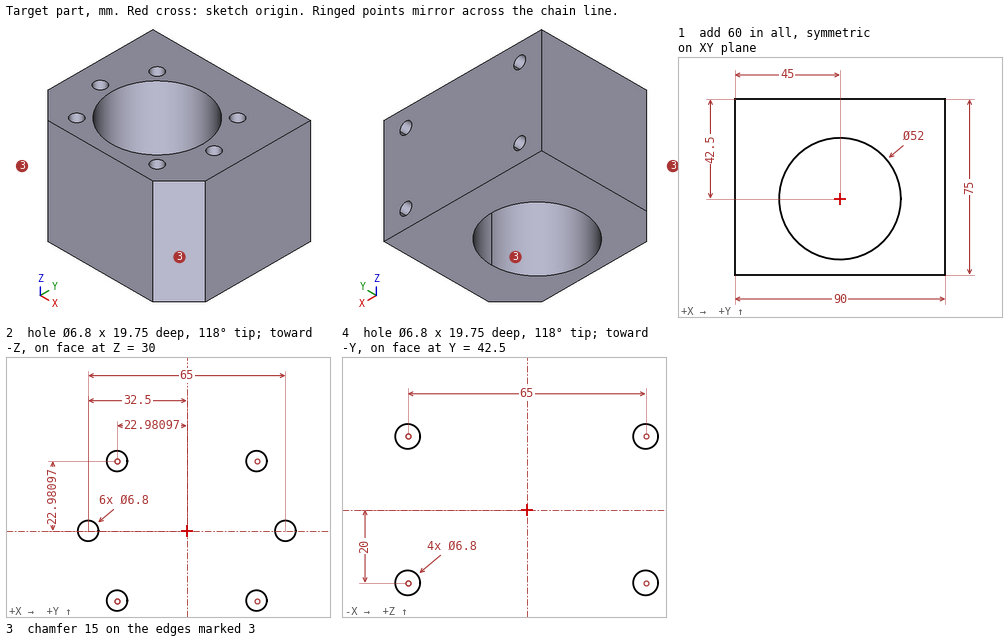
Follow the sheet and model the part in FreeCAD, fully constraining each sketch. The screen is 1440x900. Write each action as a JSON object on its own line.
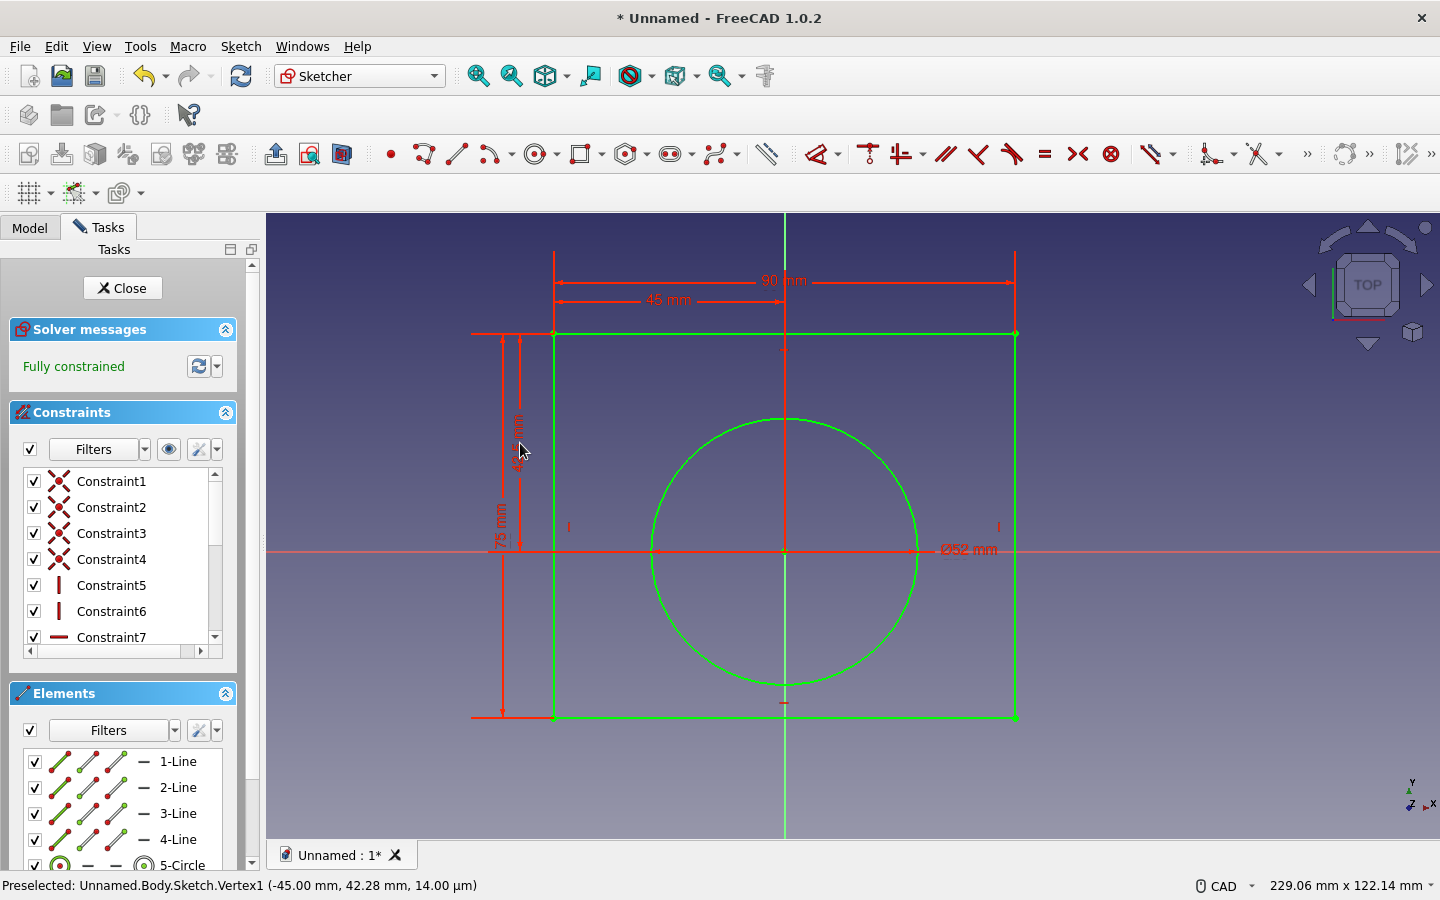
{"action": "left_click", "coordinate": [123, 288]}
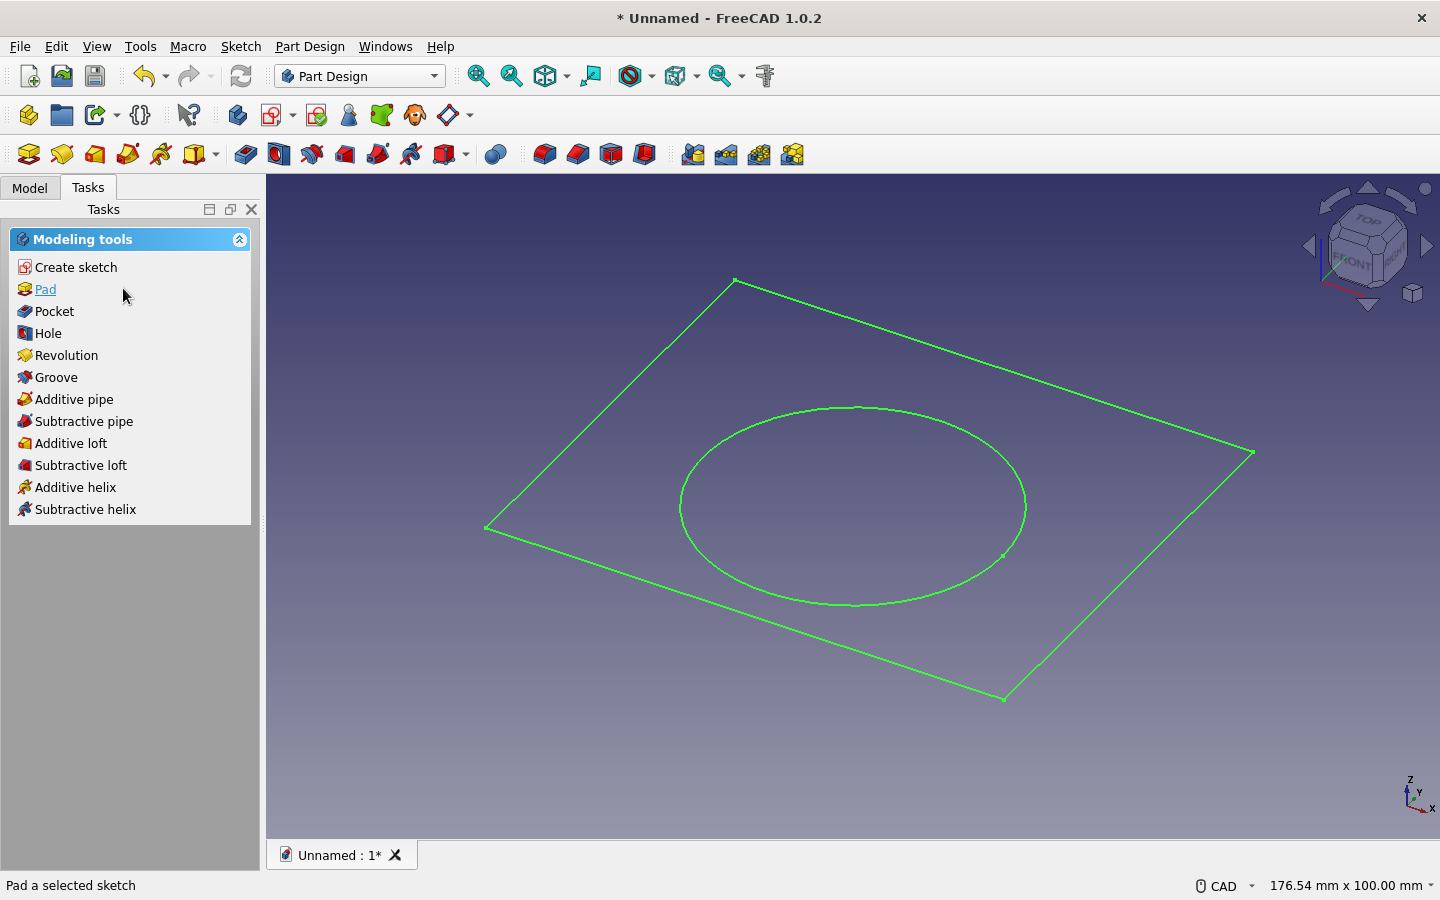
{"action": "left_click", "coordinate": [29, 154]}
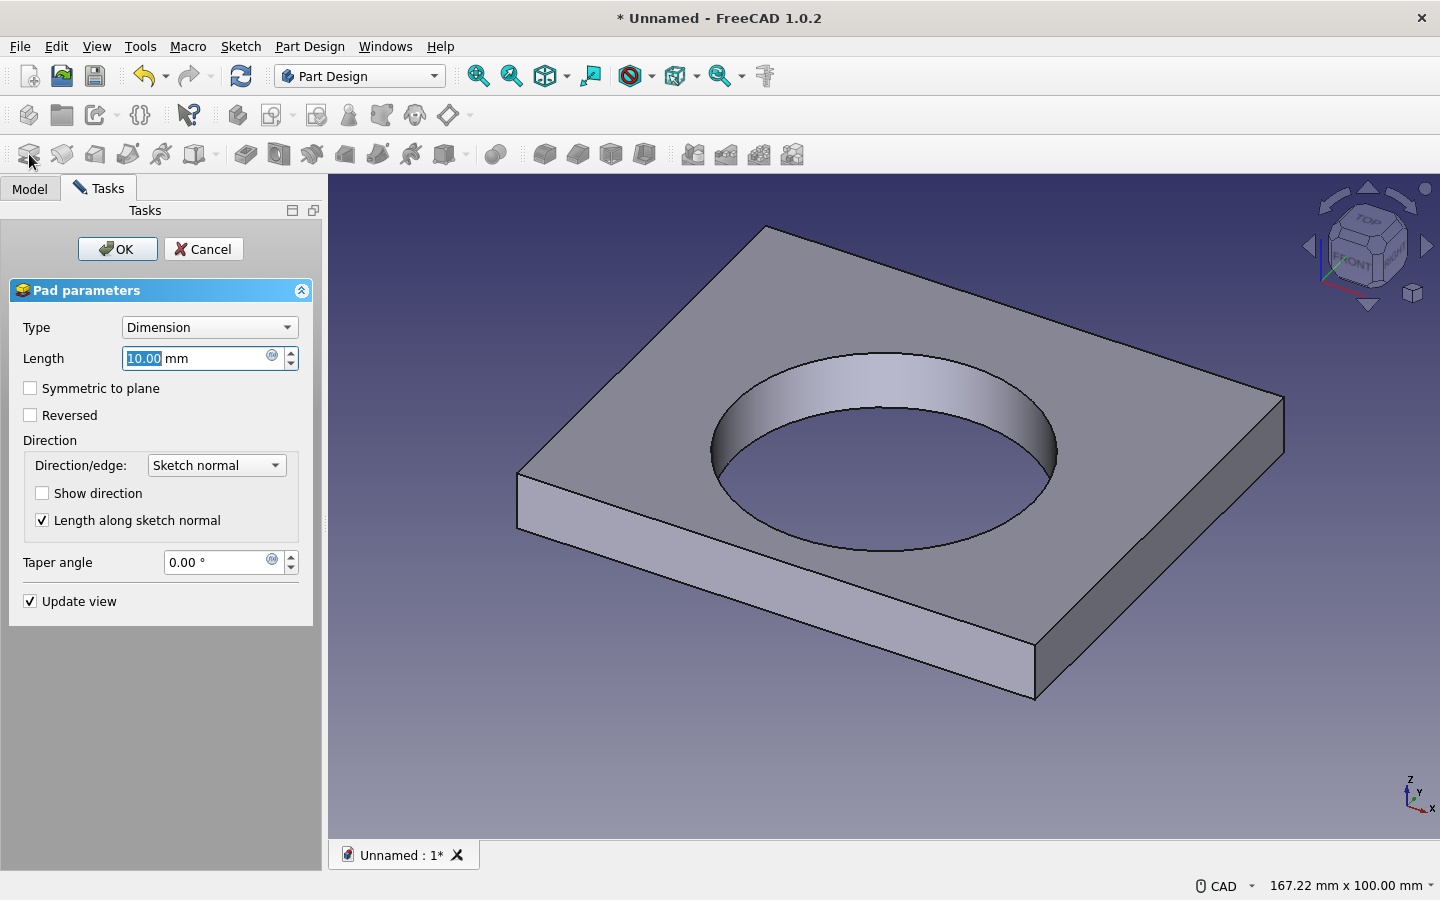
{"action": "type", "text": "60"}
{"action": "key", "text": "Tab"}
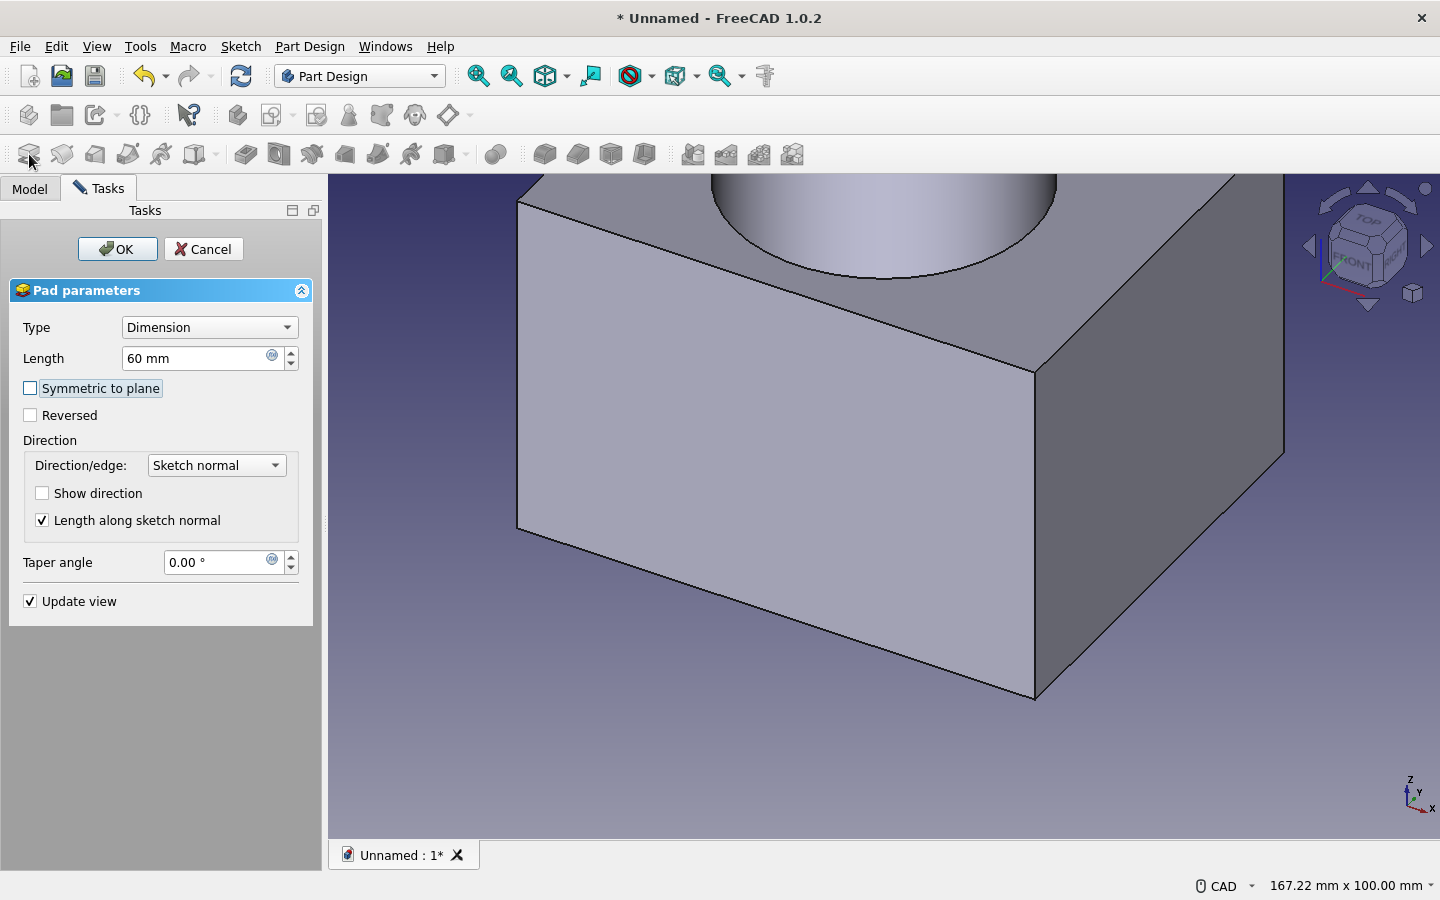
{"action": "left_click", "coordinate": [31, 388]}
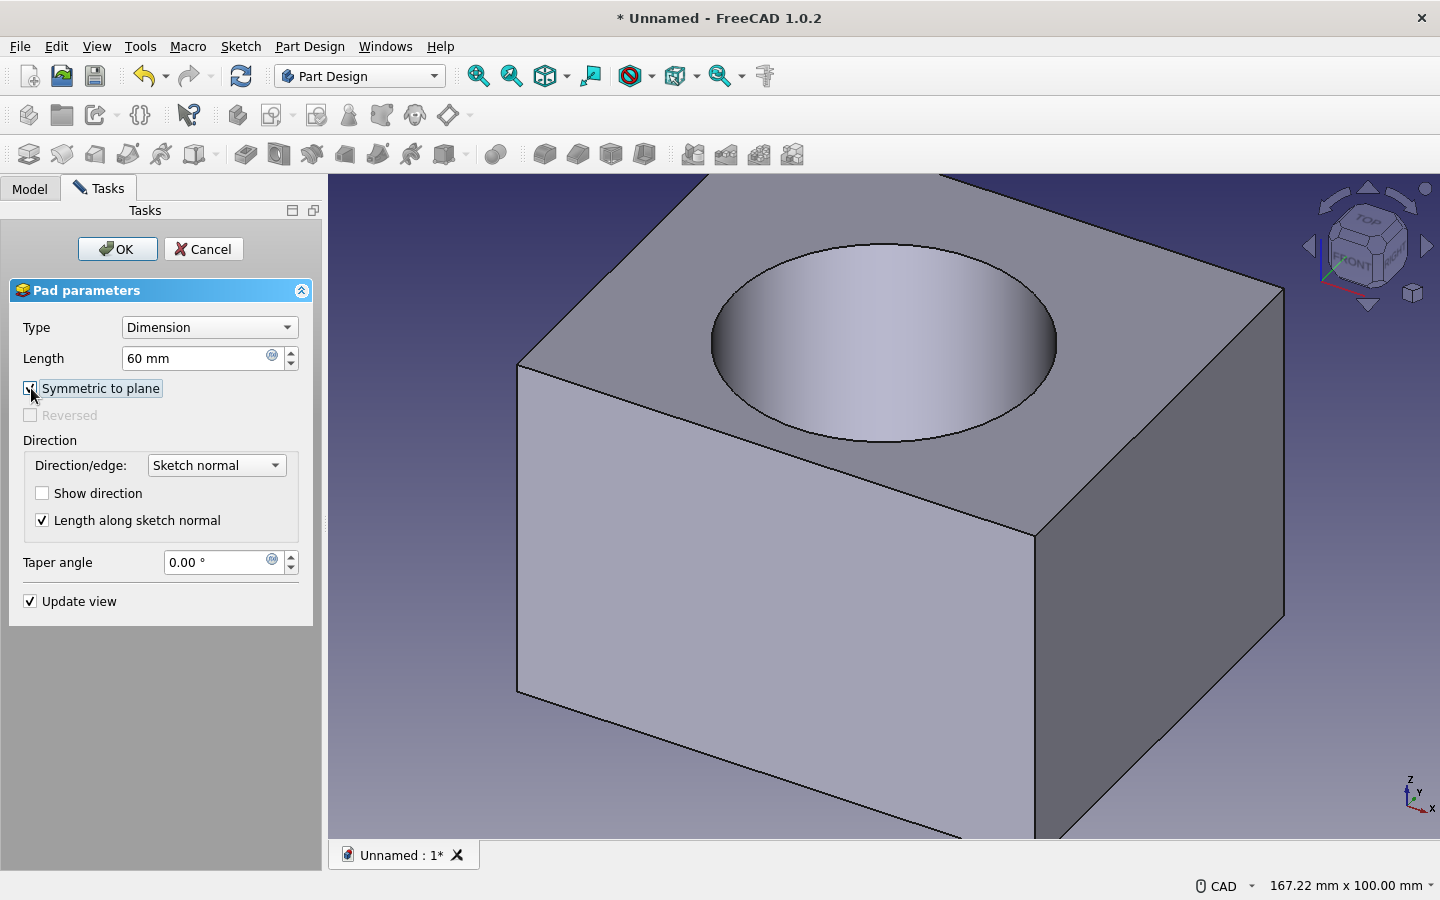
{"action": "left_click", "coordinate": [118, 249]}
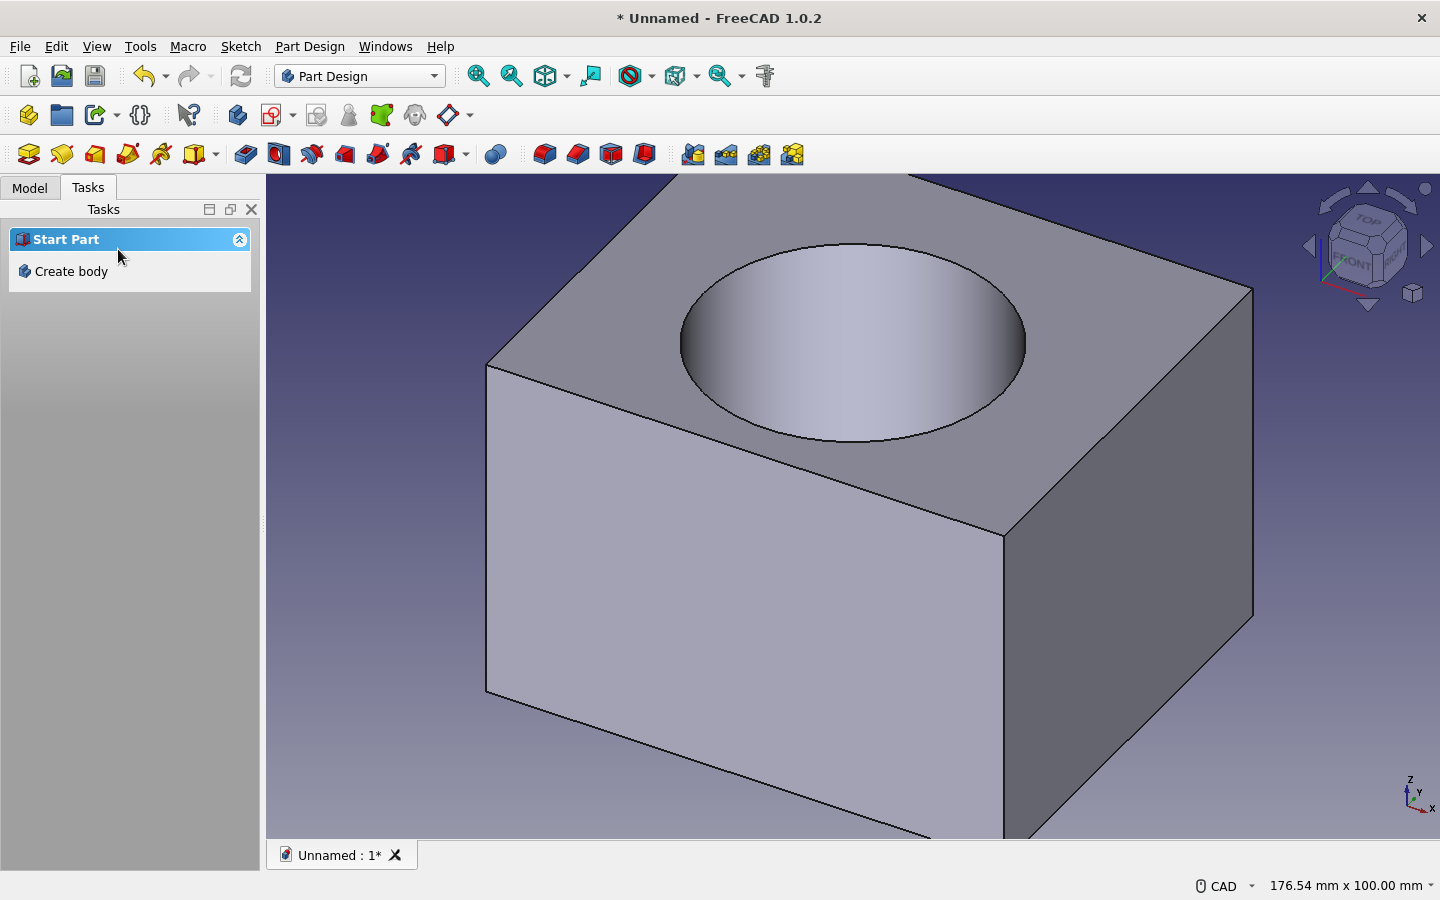
{"action": "left_click", "coordinate": [479, 76]}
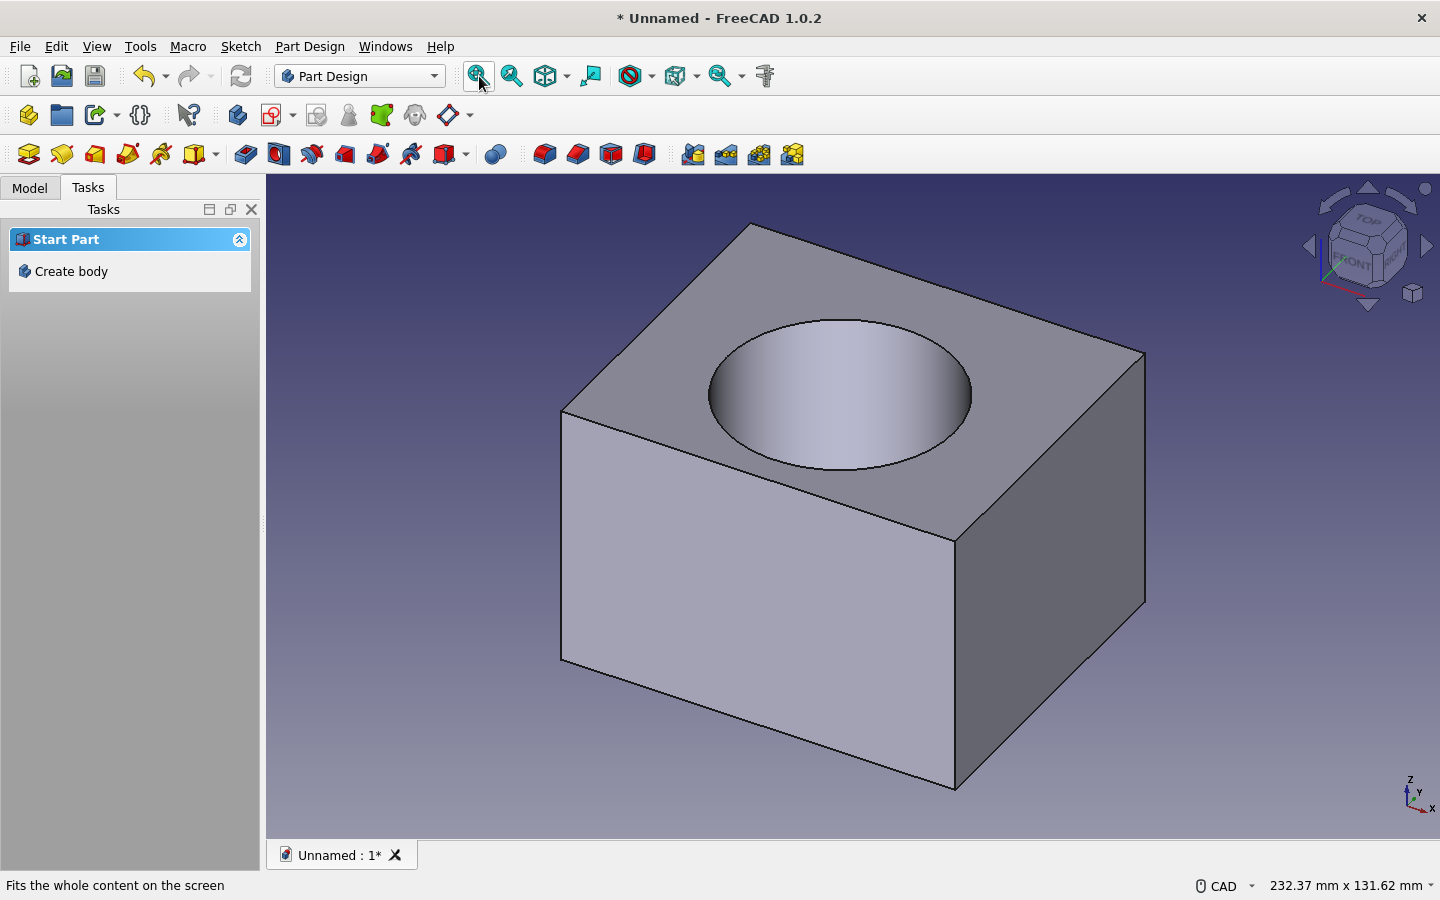
{"action": "left_click", "coordinate": [795, 290]}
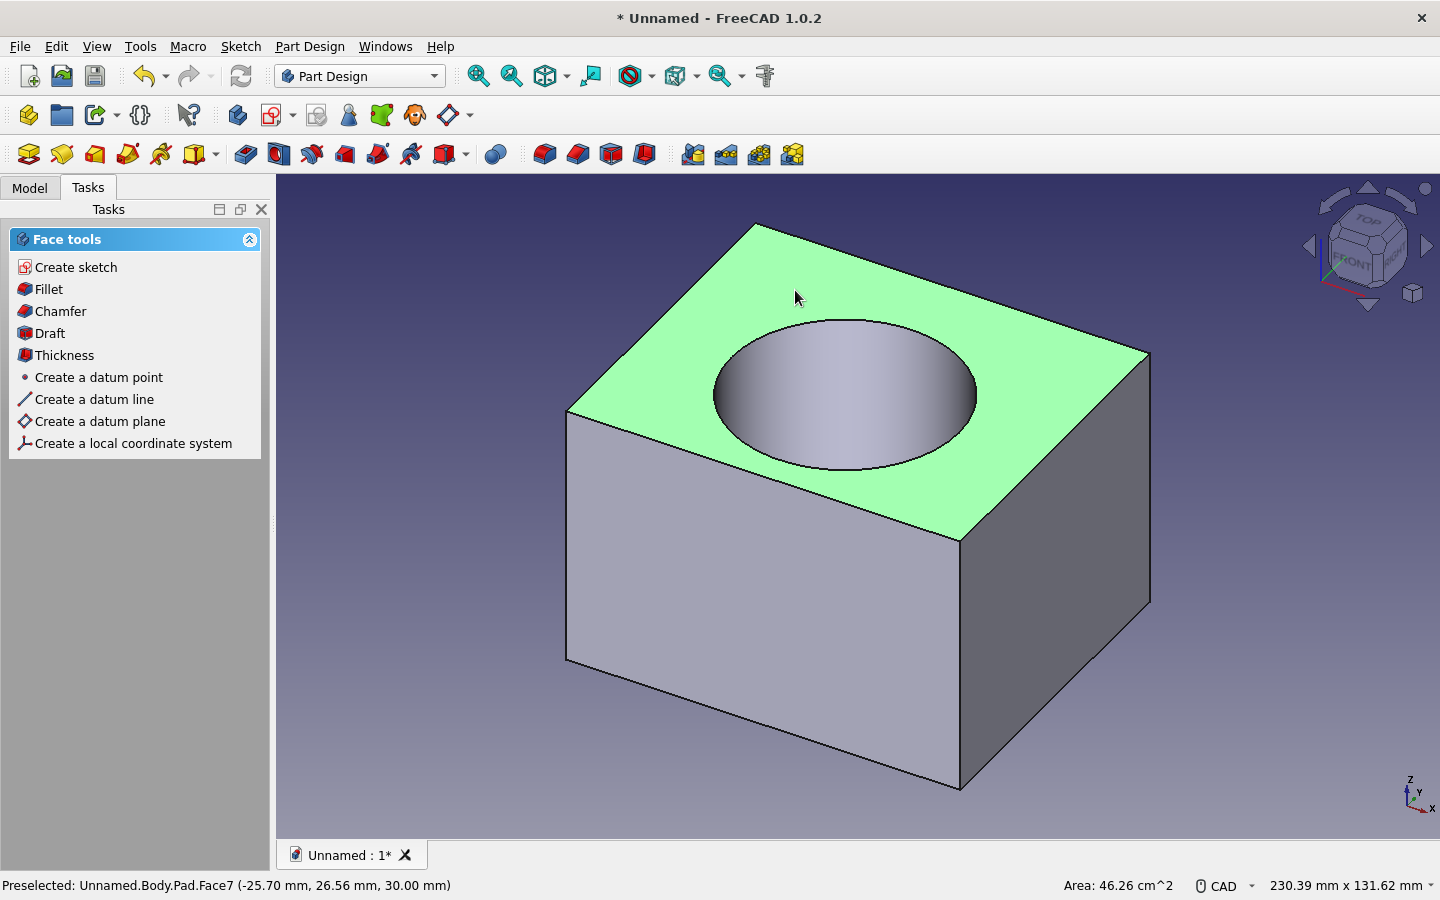
{"action": "left_click", "coordinate": [270, 116]}